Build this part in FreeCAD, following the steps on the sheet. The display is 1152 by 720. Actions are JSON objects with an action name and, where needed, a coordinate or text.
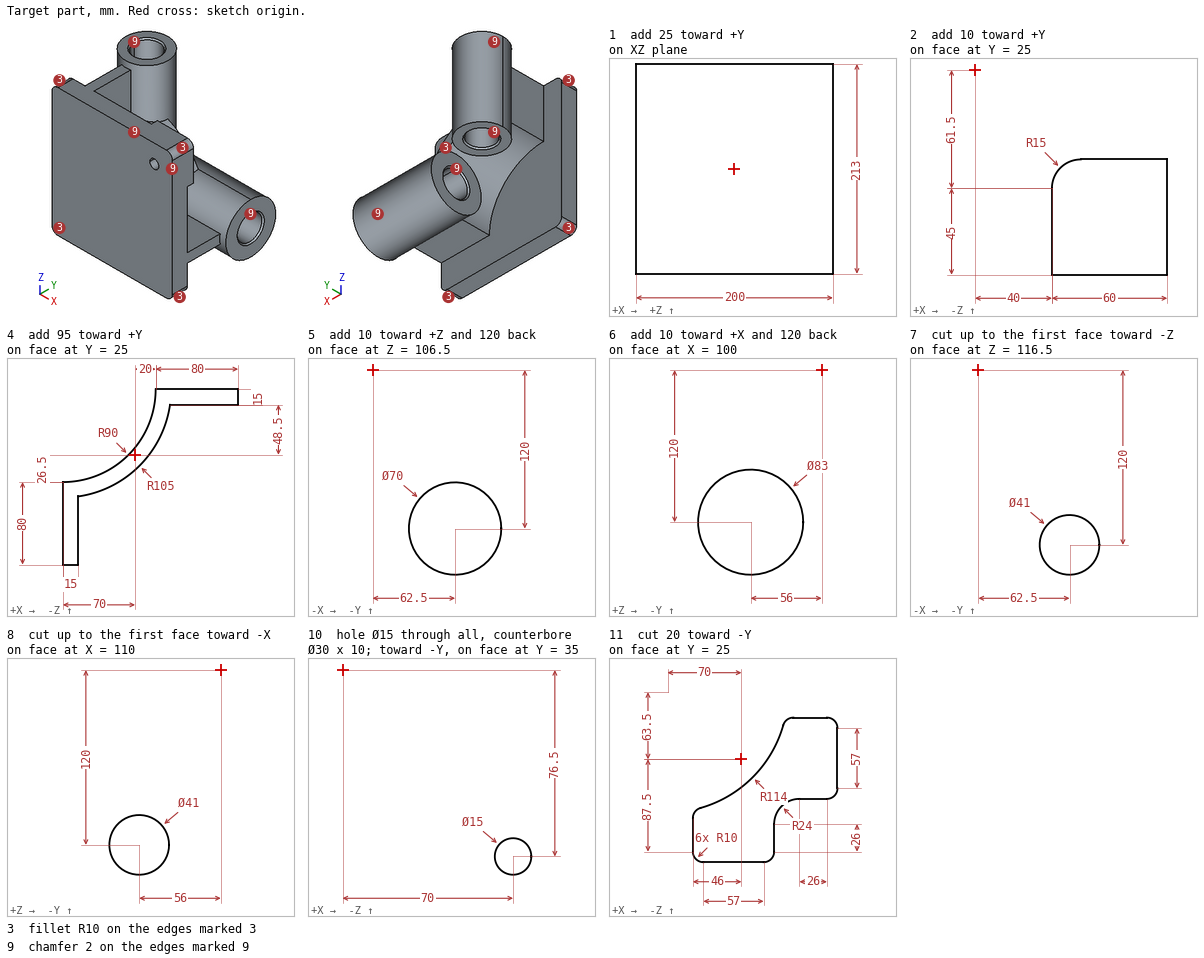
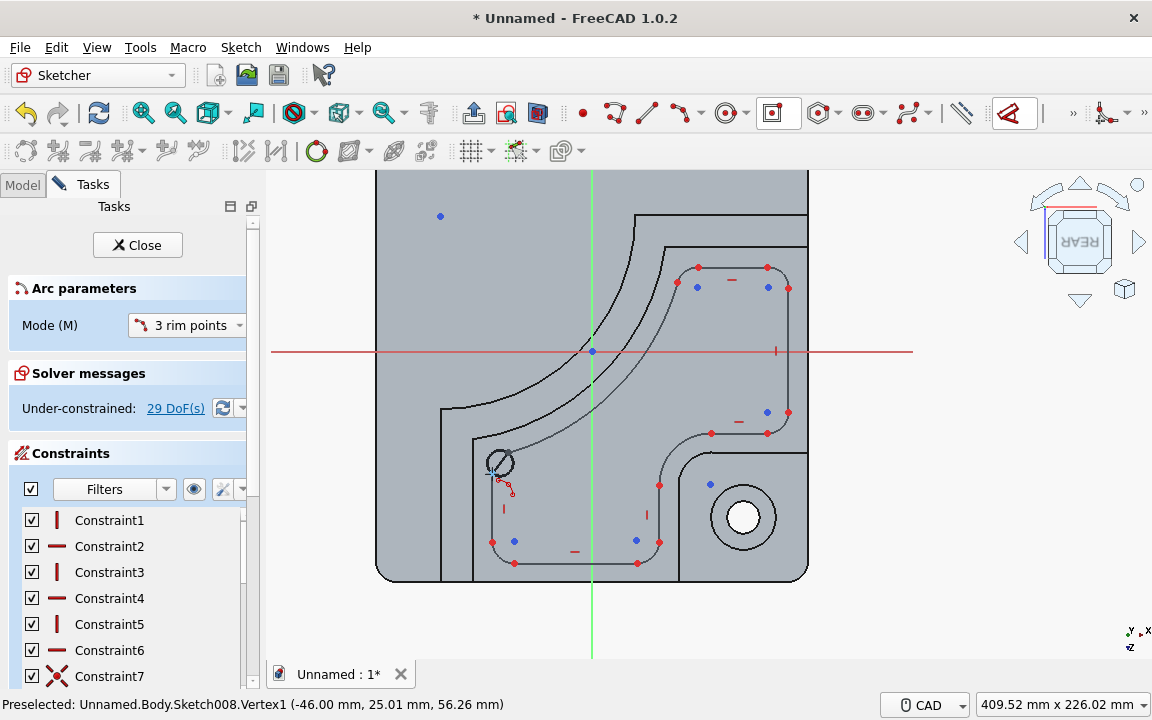
{"action": "scroll", "coordinate": [497, 459], "scroll_direction": "up", "scroll_amount": 7}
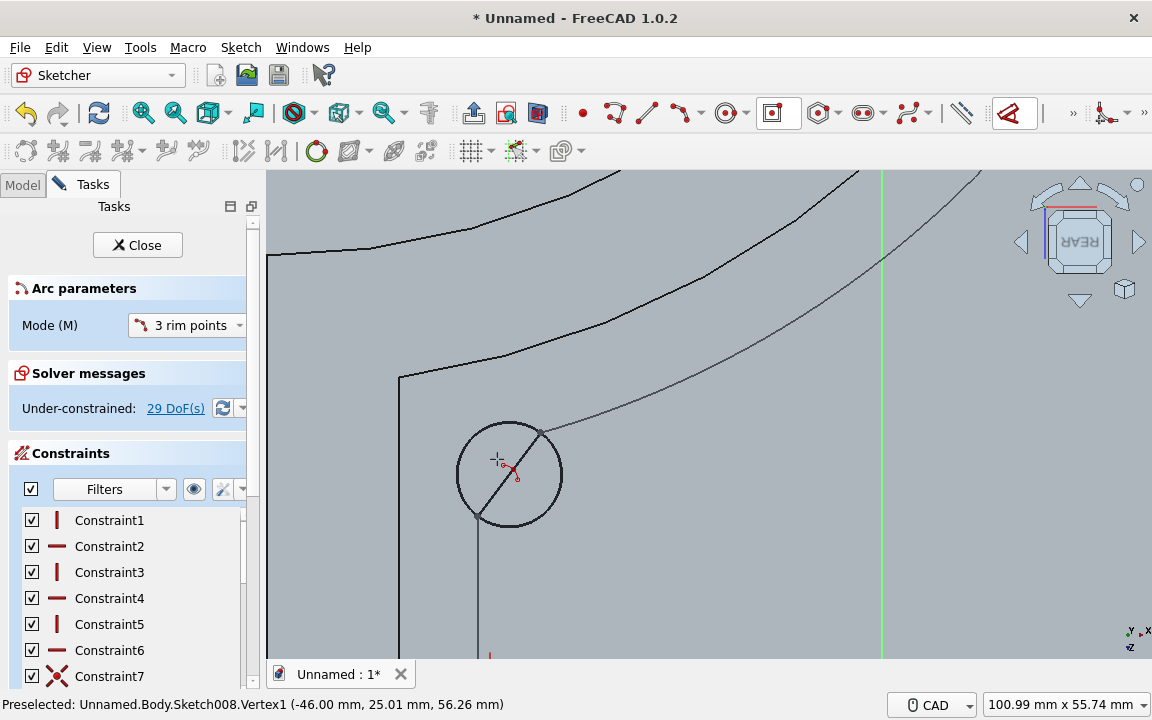
{"action": "left_click", "coordinate": [496, 459]}
{"action": "key", "text": "Escape"}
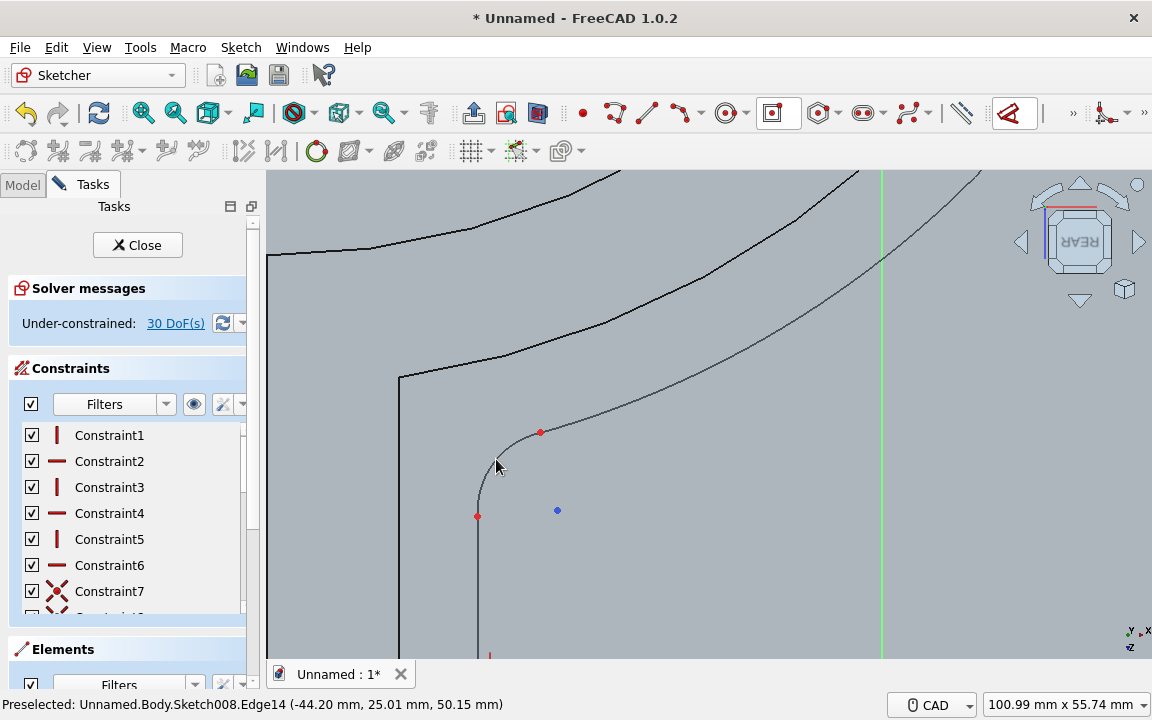
{"action": "scroll", "coordinate": [497, 459], "scroll_direction": "down", "scroll_amount": 7}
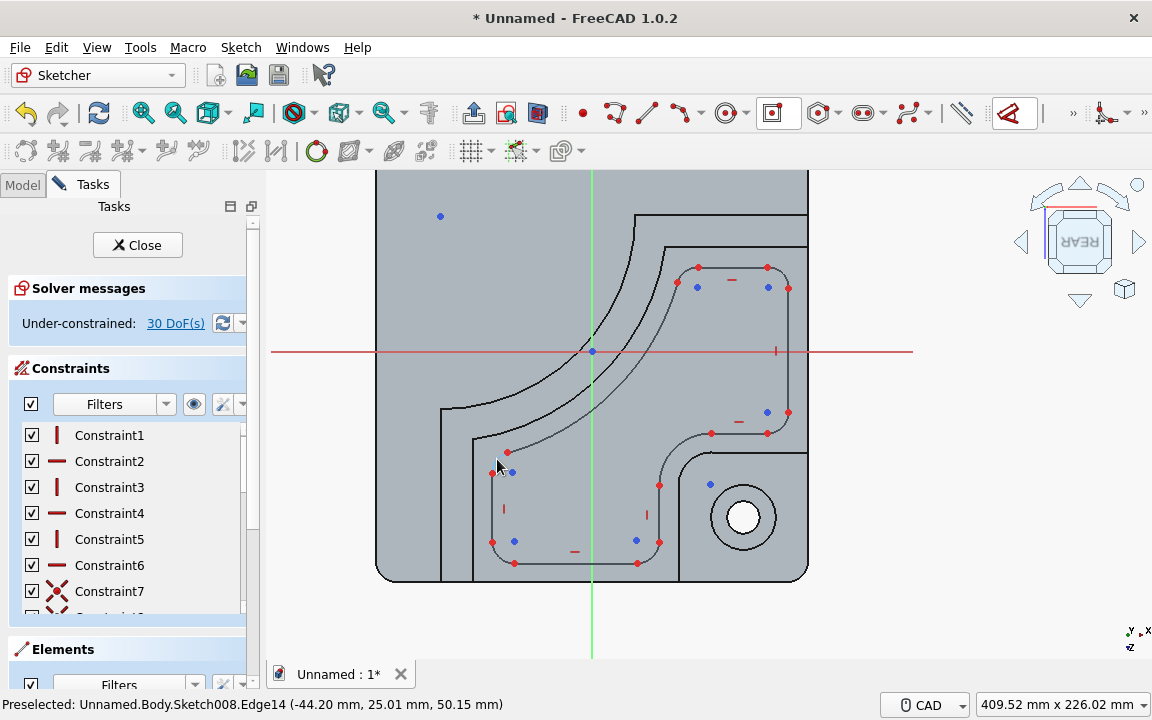
{"action": "left_click", "coordinate": [492, 494]}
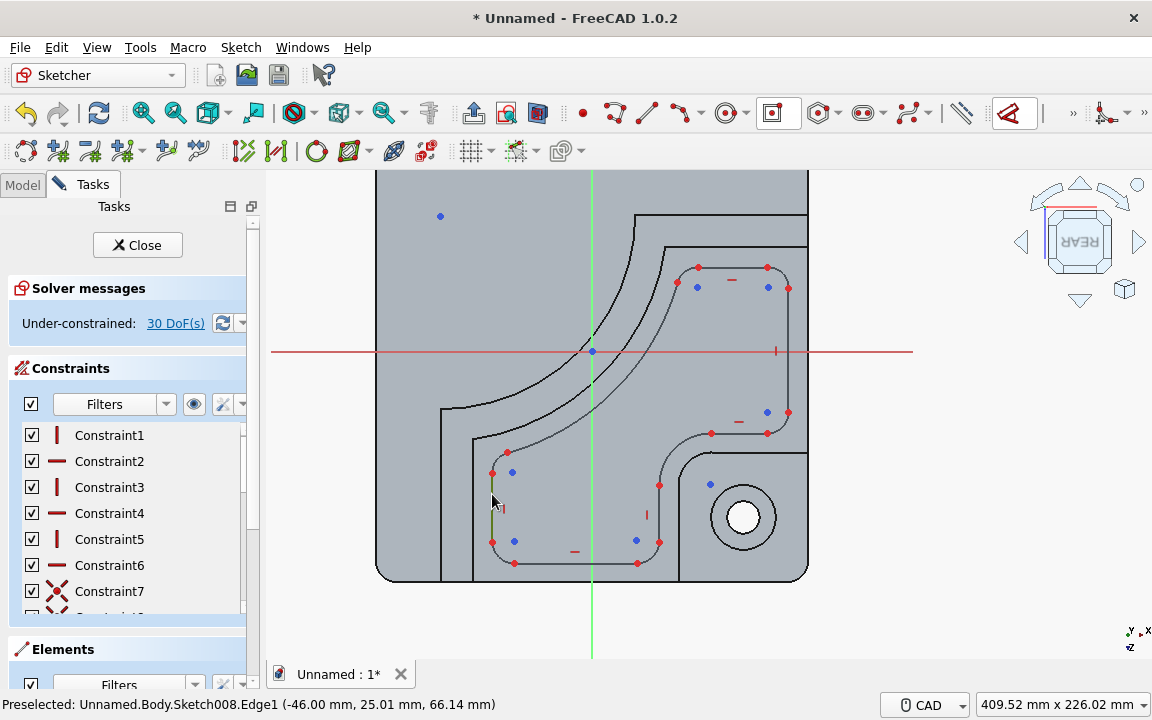
{"action": "scroll", "coordinate": [495, 552], "scroll_direction": "up", "scroll_amount": 2}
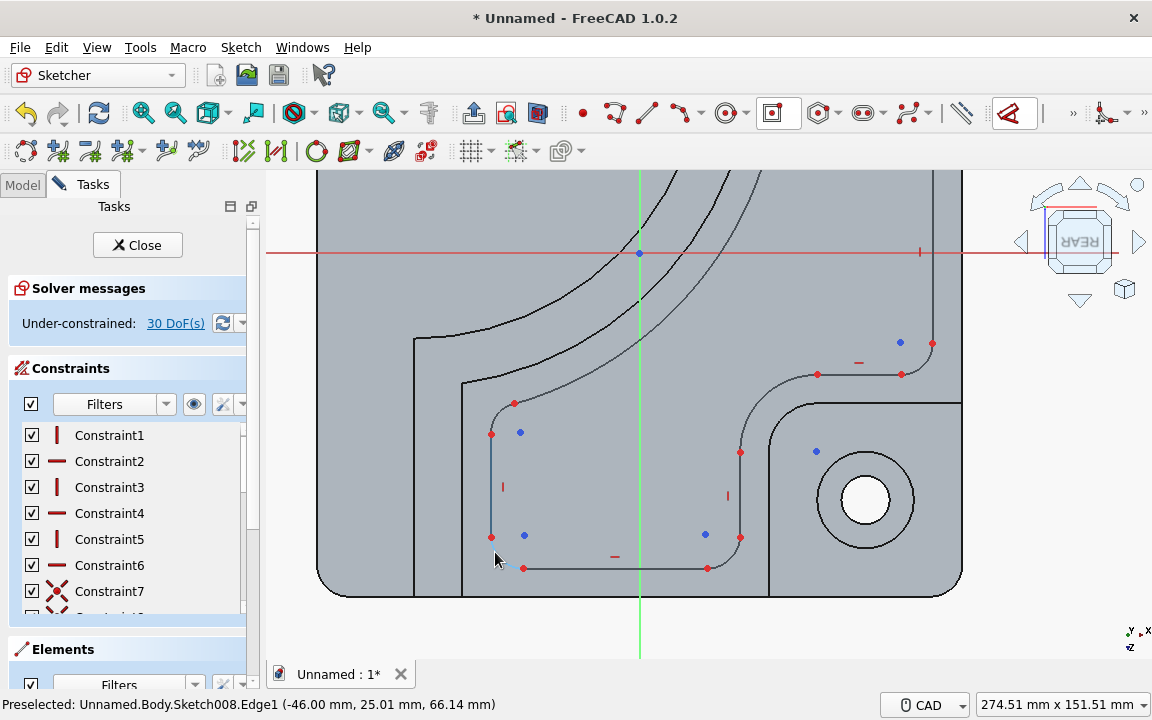
{"action": "left_click", "coordinate": [495, 552]}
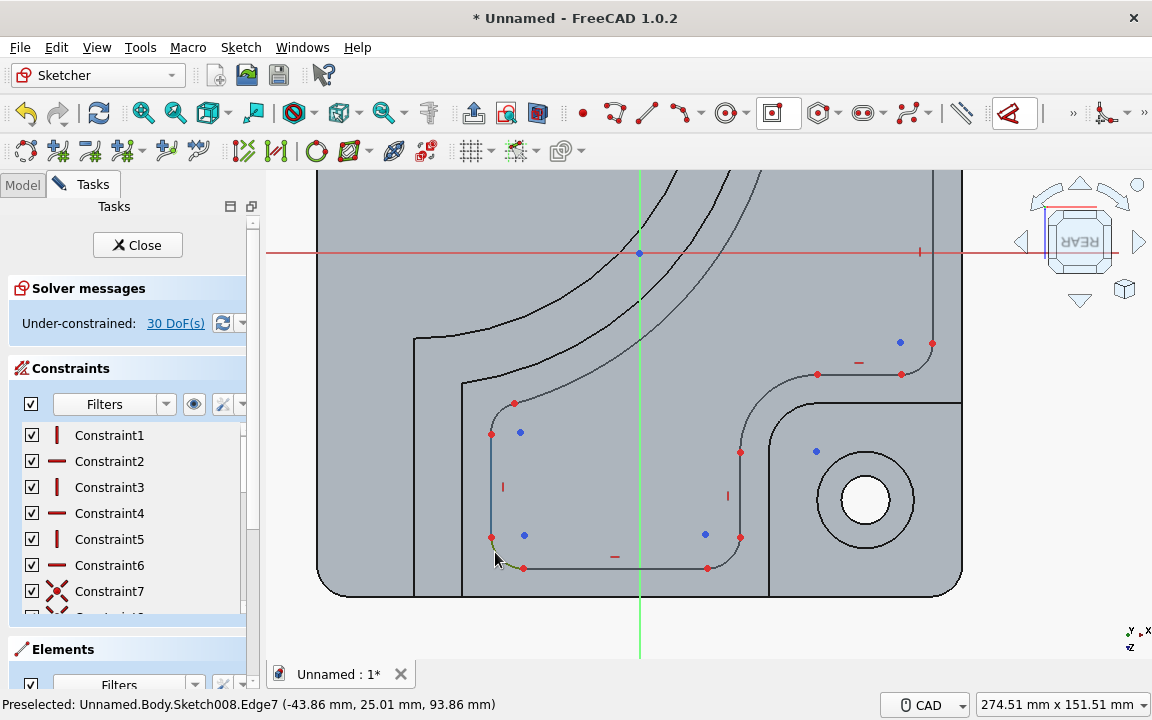
{"action": "key", "text": "t"}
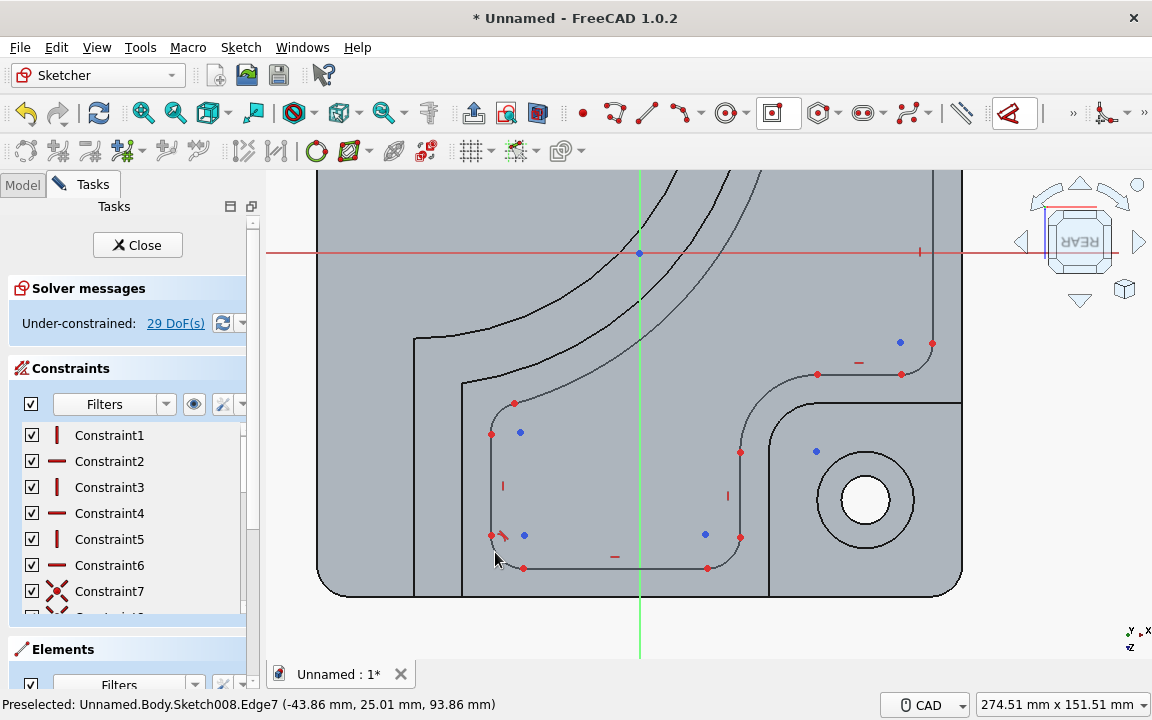
{"action": "left_click", "coordinate": [491, 465]}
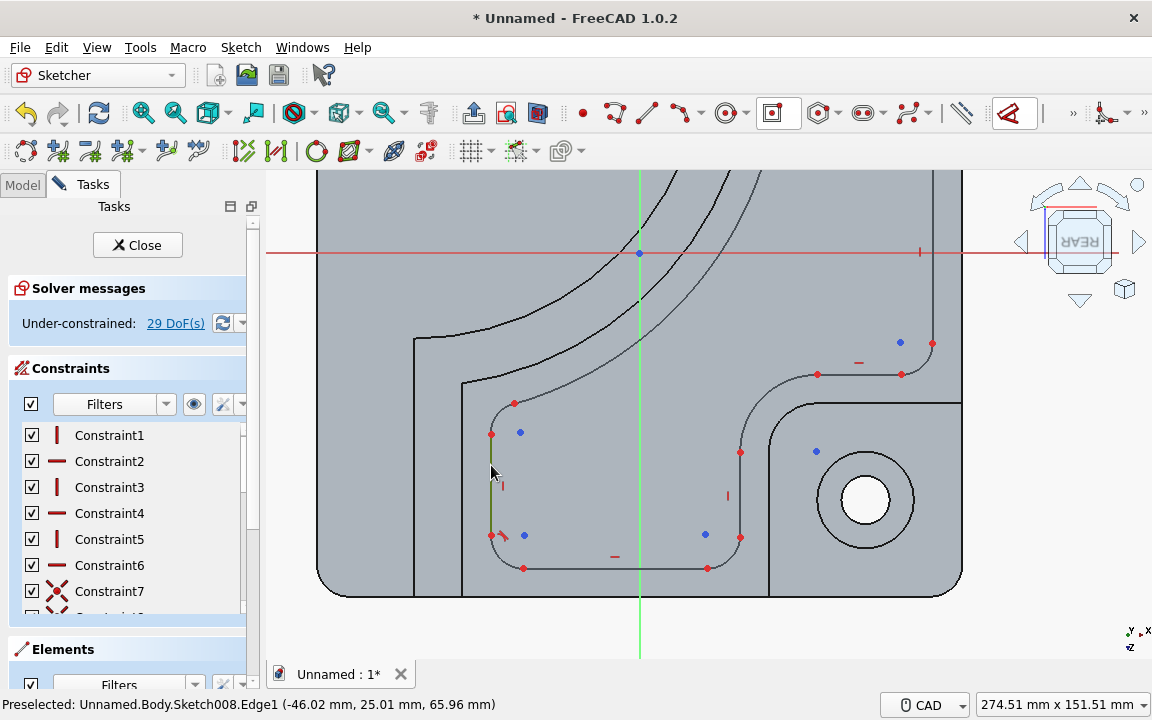
{"action": "left_click", "coordinate": [503, 409]}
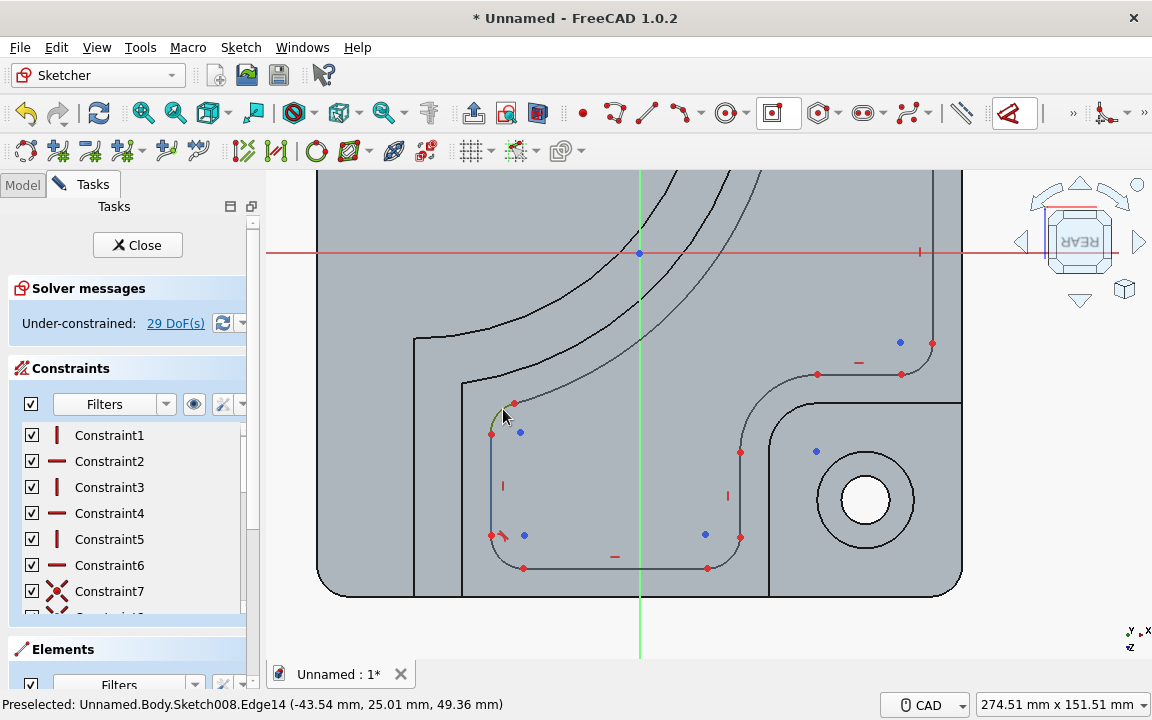
{"action": "key", "text": "t"}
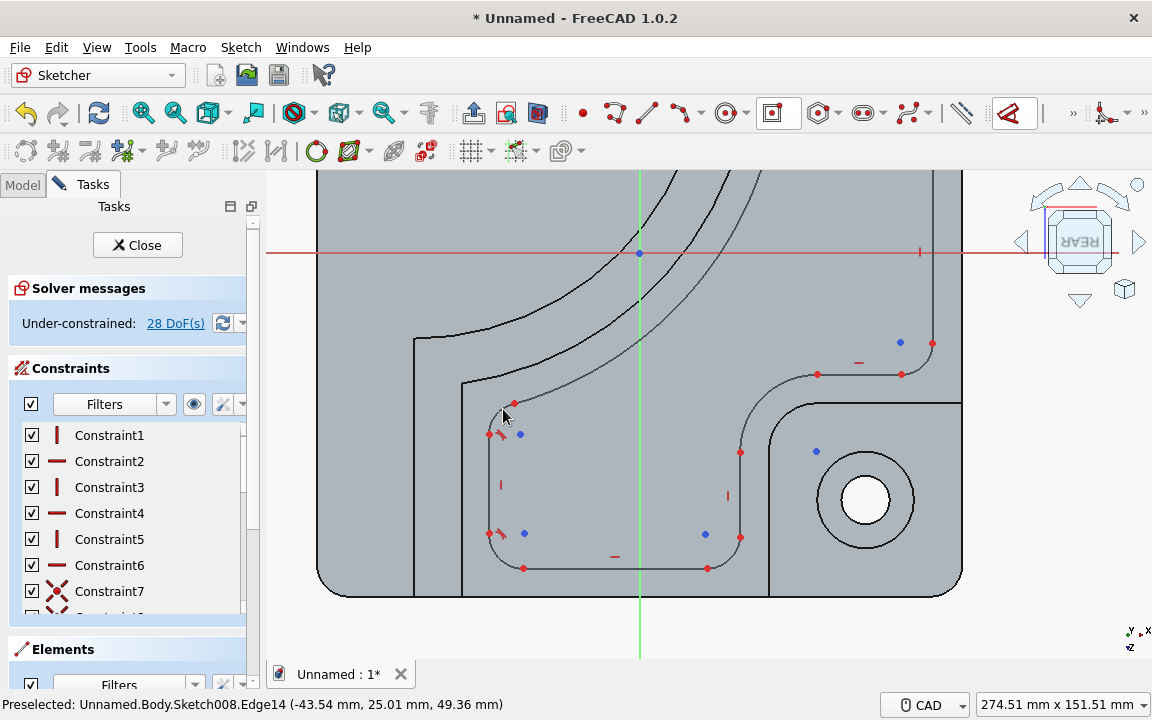
{"action": "left_click", "coordinate": [579, 569]}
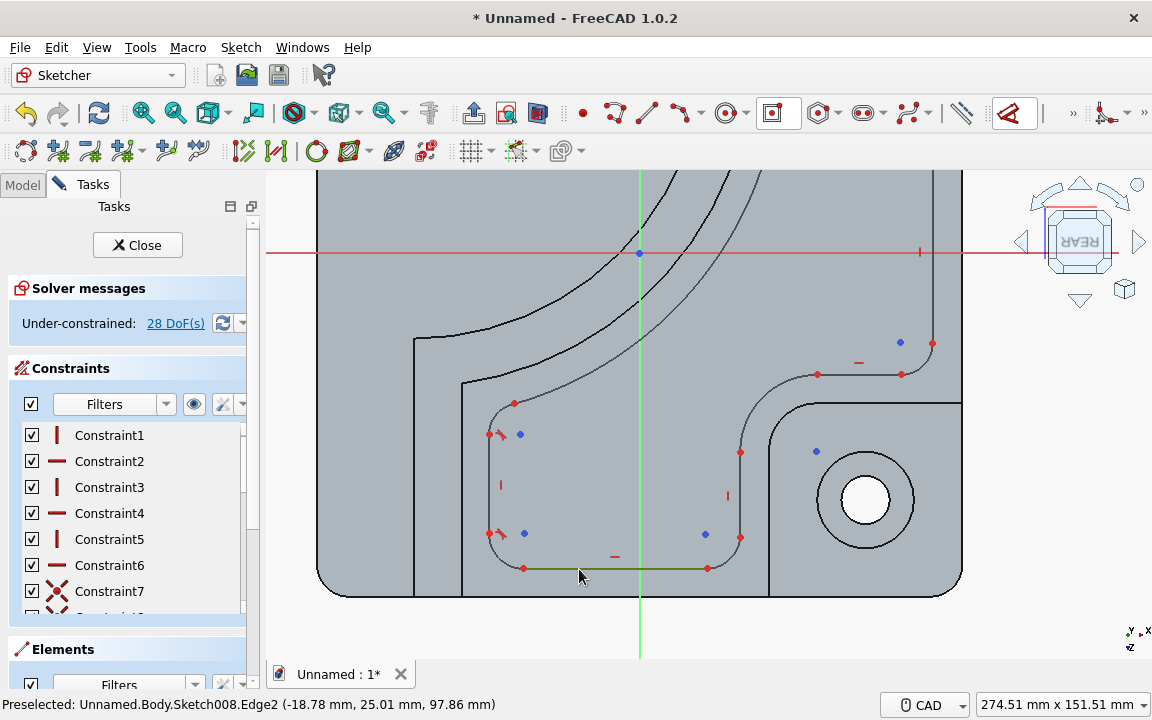
{"action": "left_click", "coordinate": [493, 550]}